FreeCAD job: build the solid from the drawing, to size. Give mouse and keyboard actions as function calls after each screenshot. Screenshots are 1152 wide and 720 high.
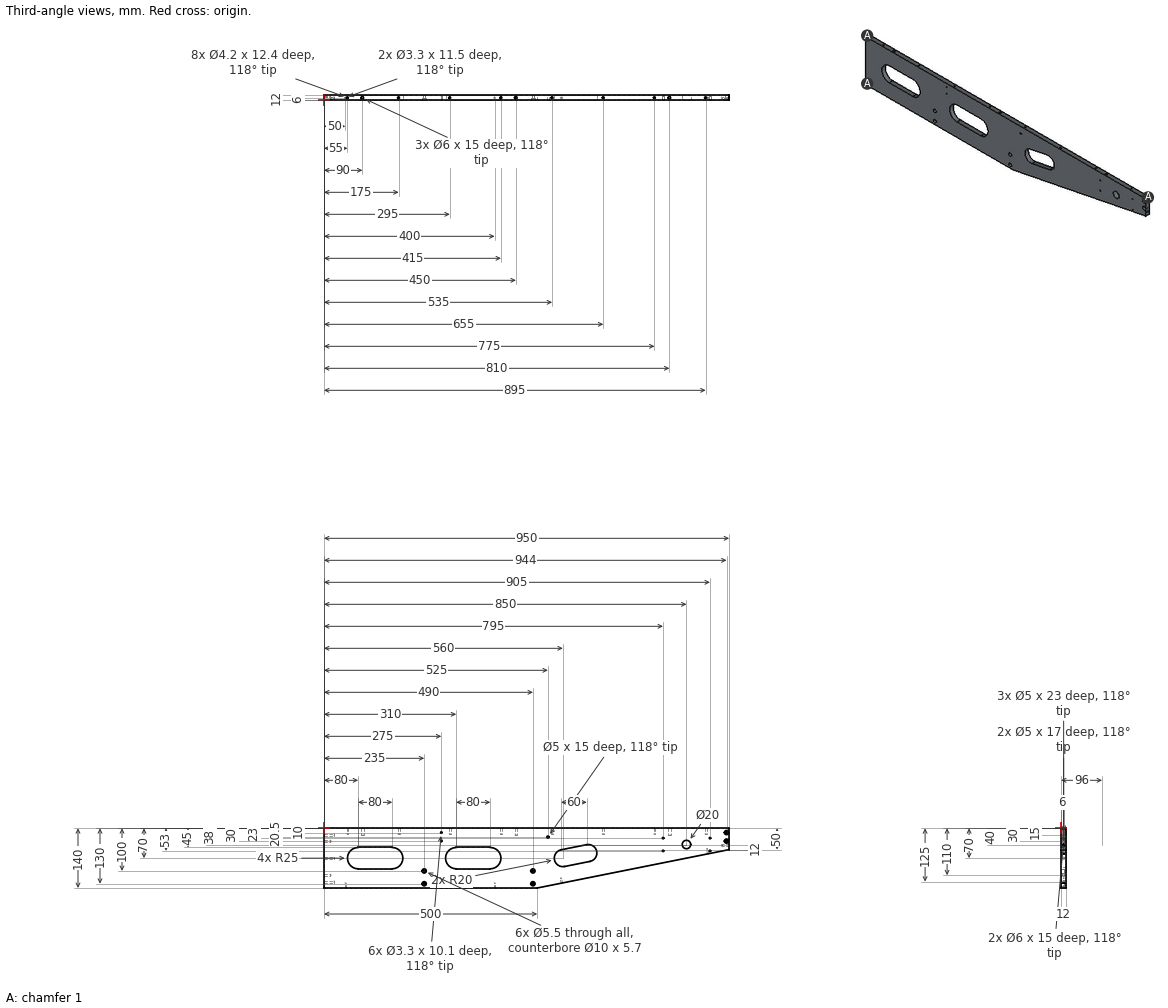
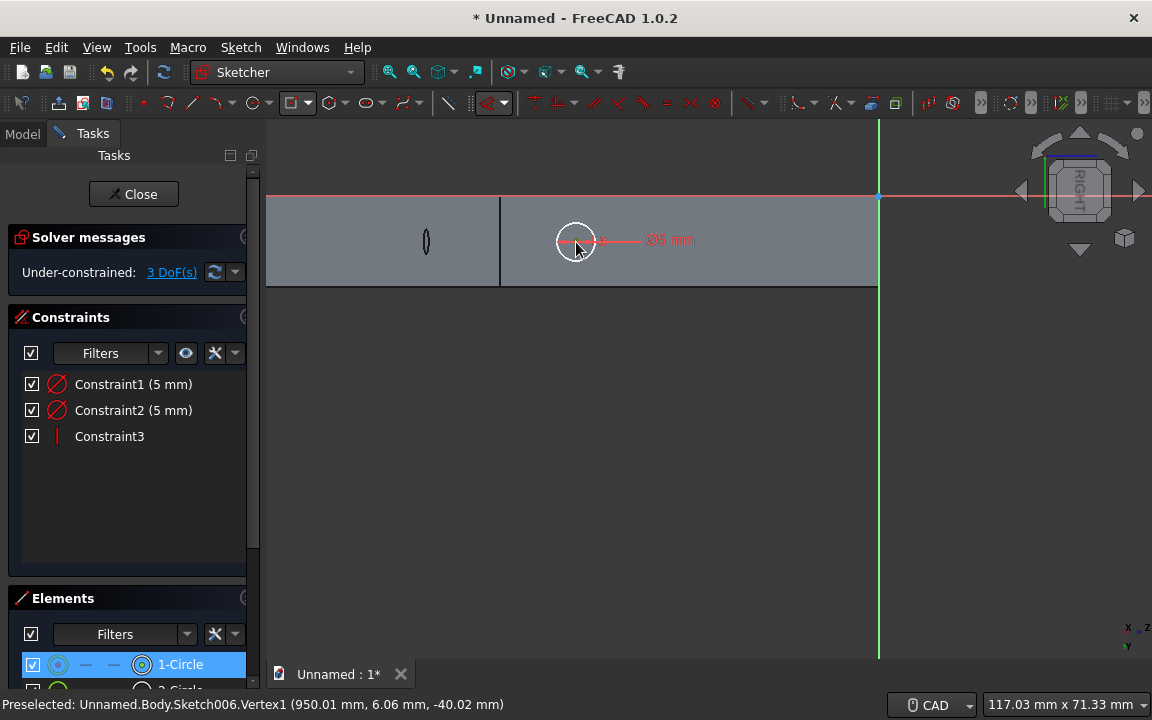
key(i)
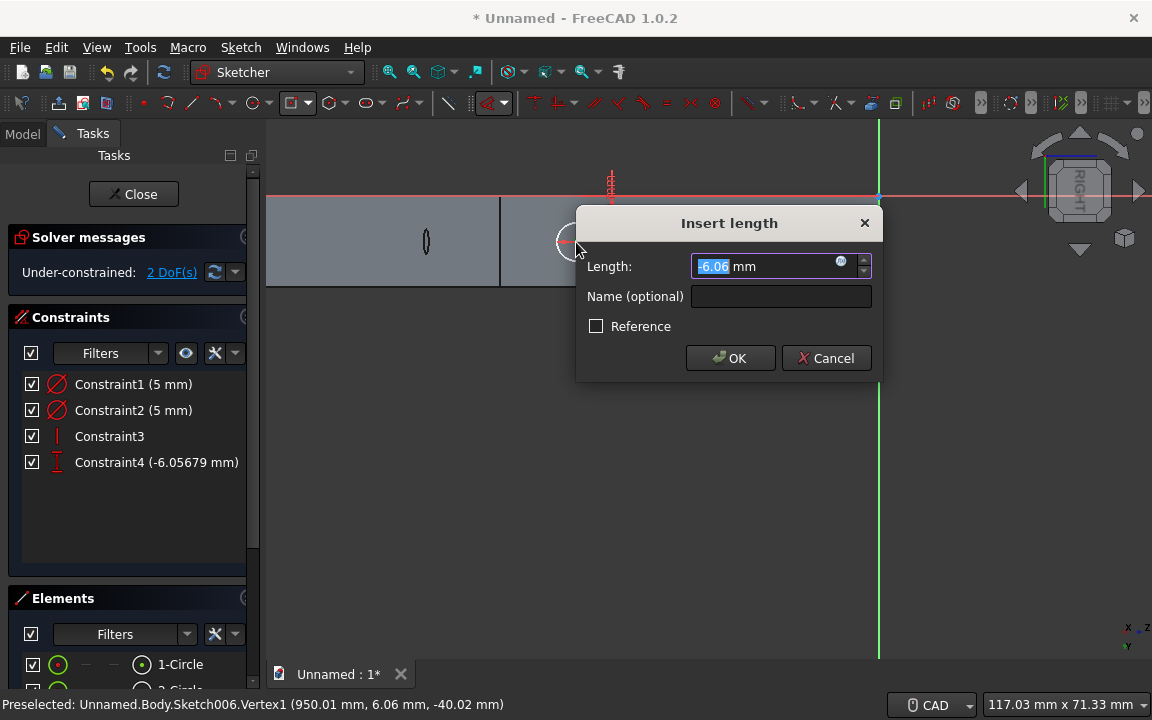
text(-6)
key(Return)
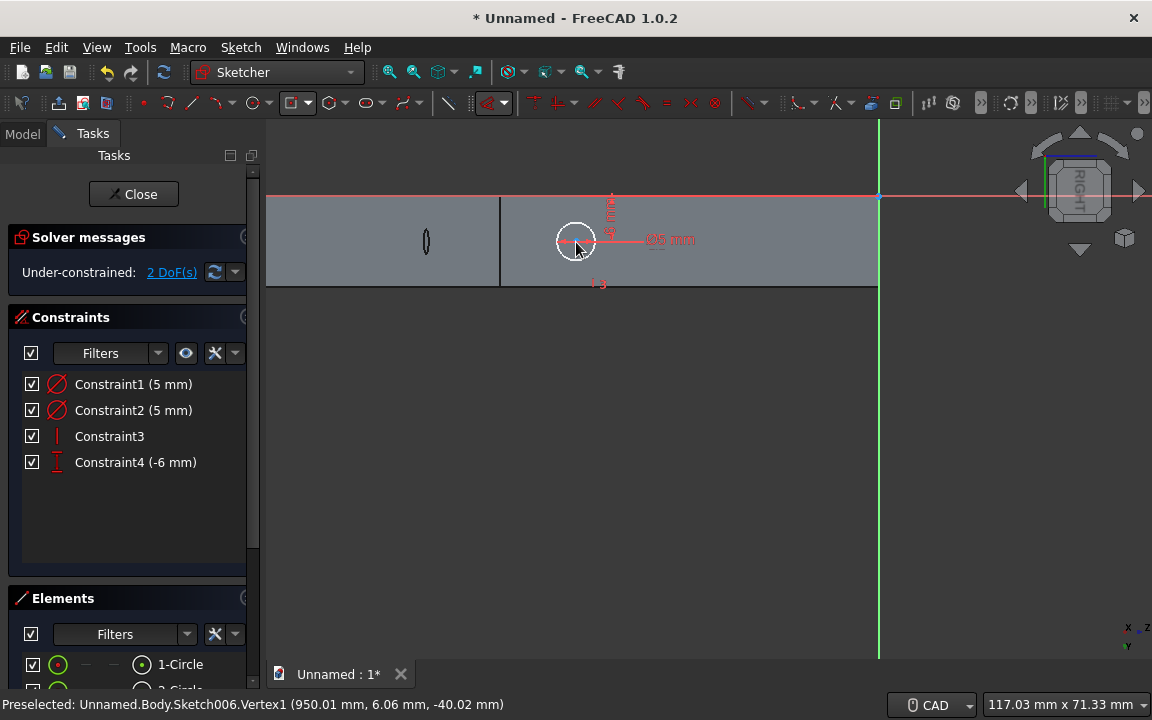
click(576, 242)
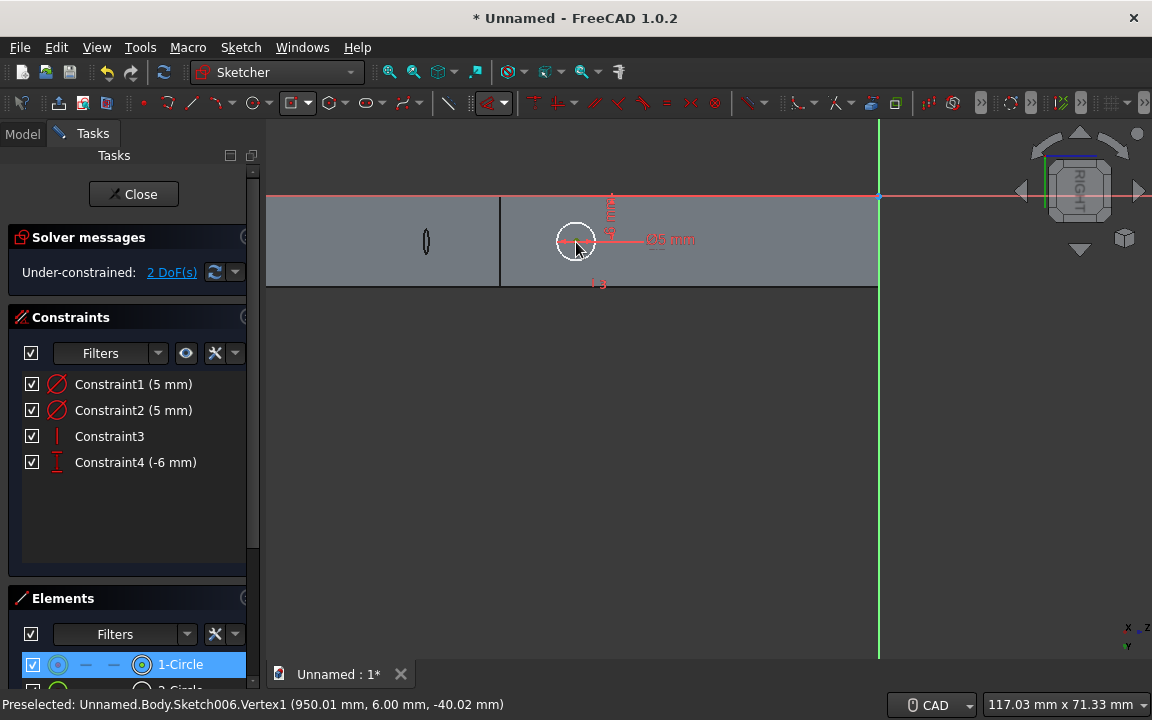
click(506, 104)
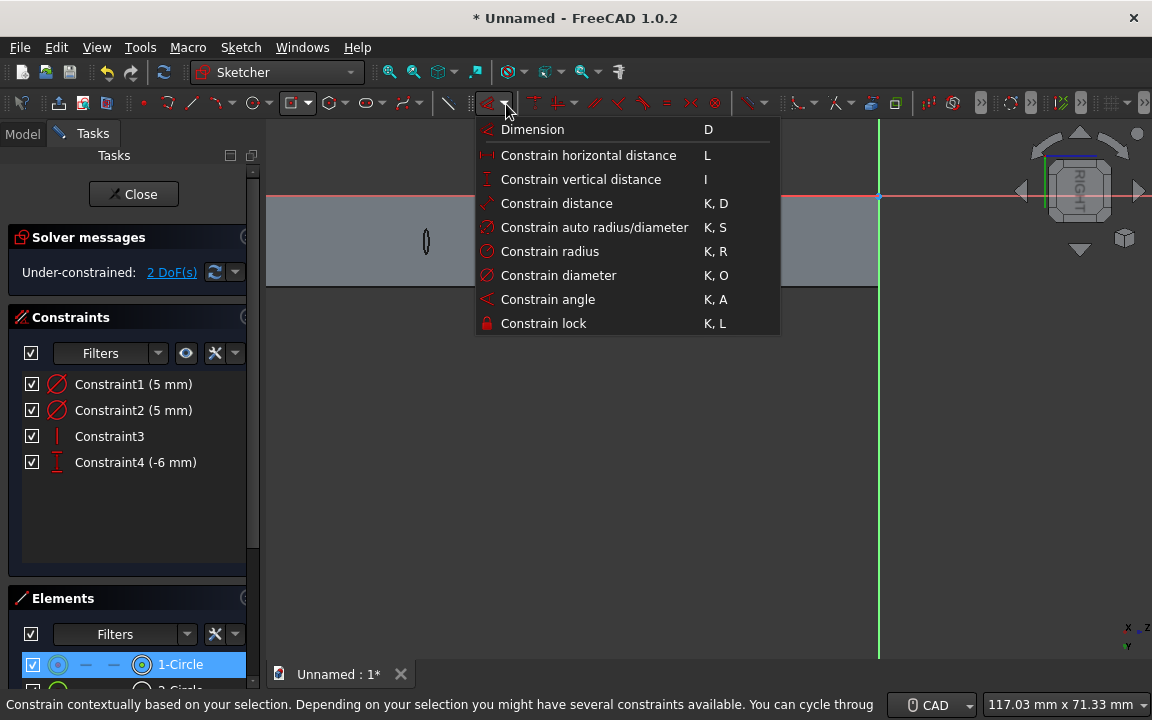
click(628, 155)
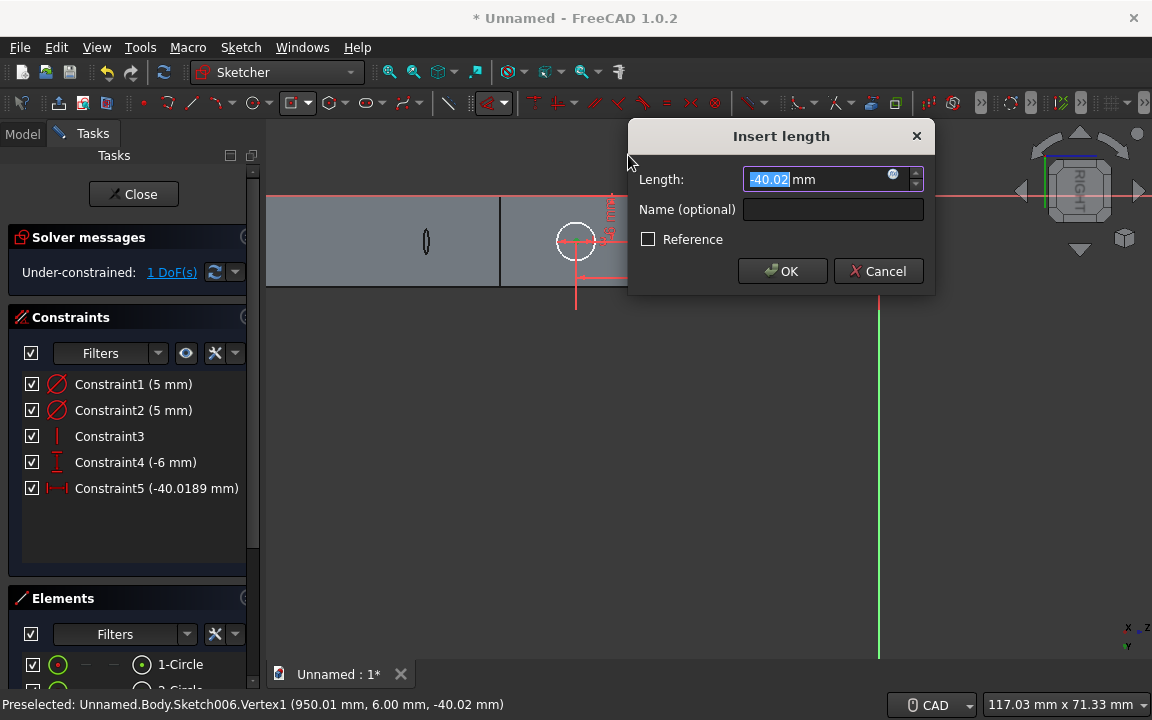
text(-40)
key(Return)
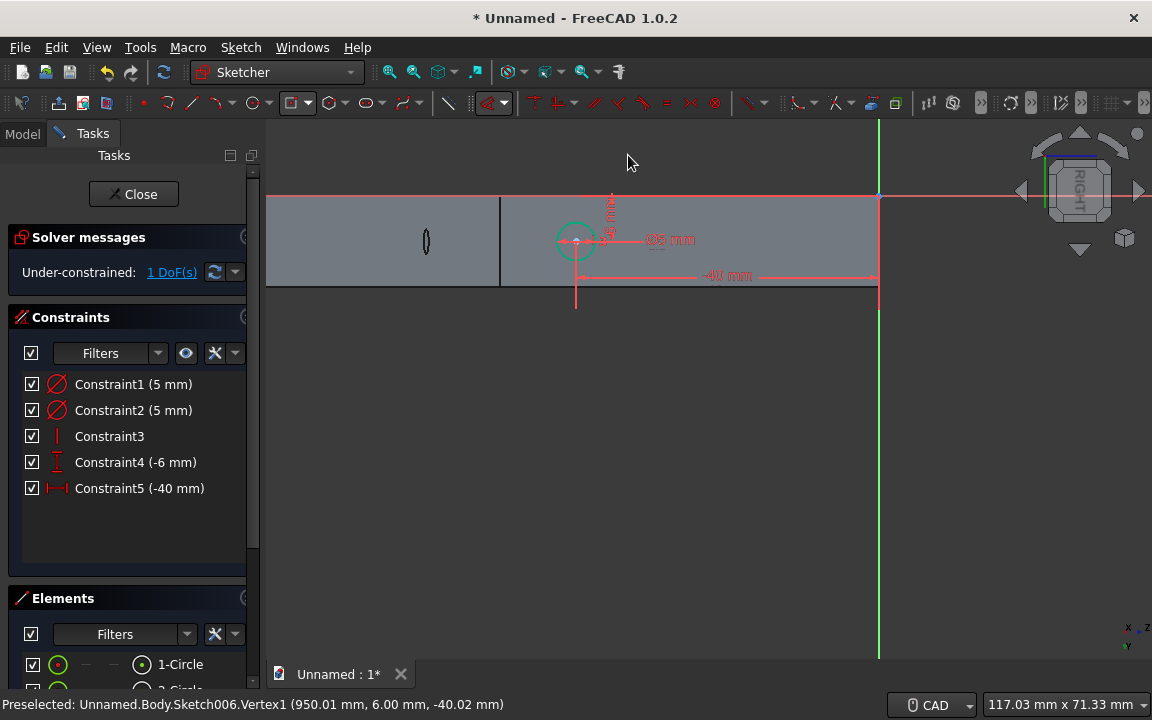
scroll(577, 242, down, 4)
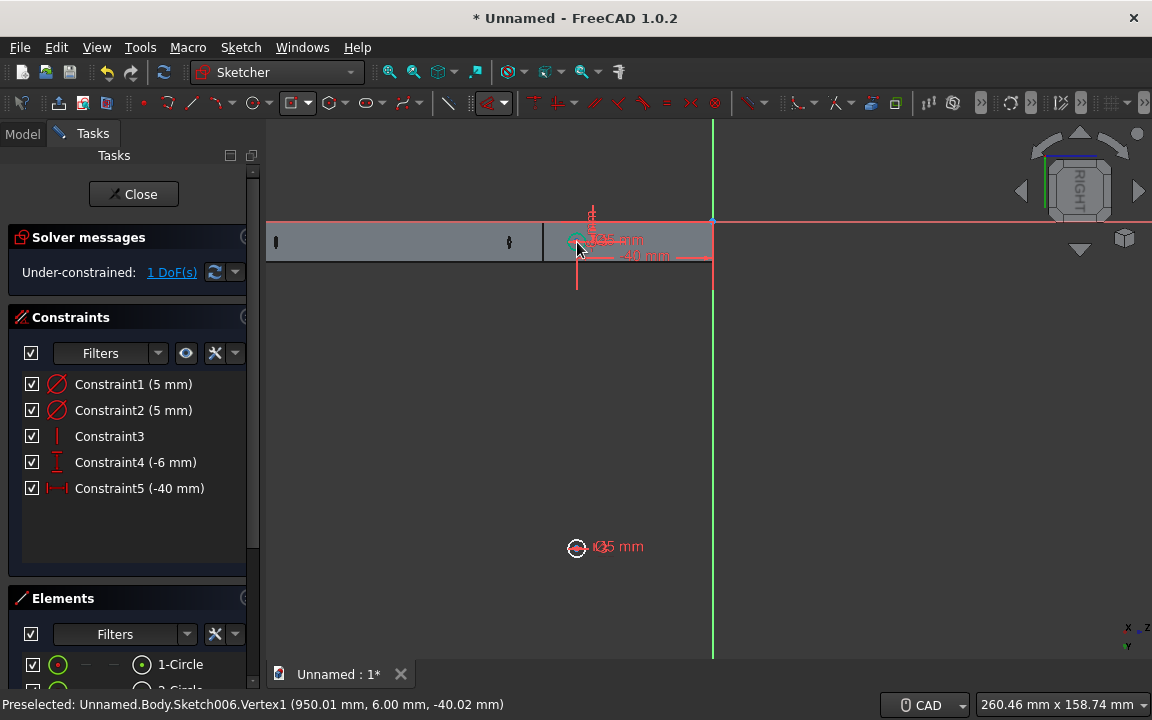
click(577, 549)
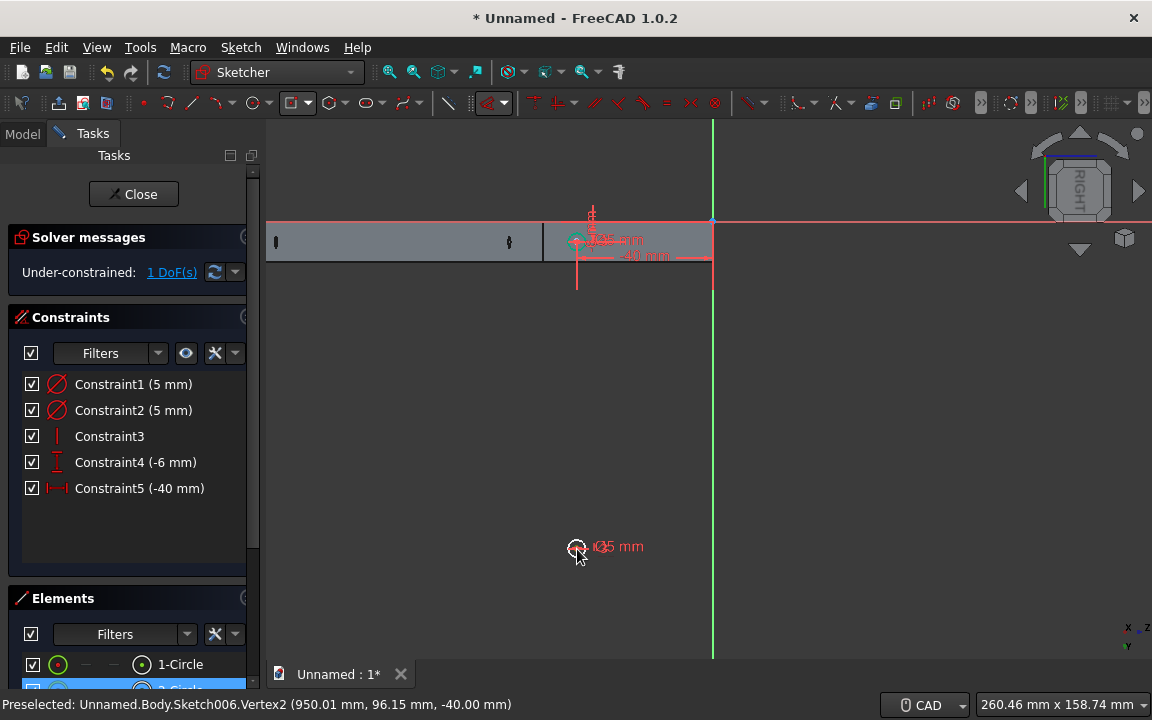
key(i)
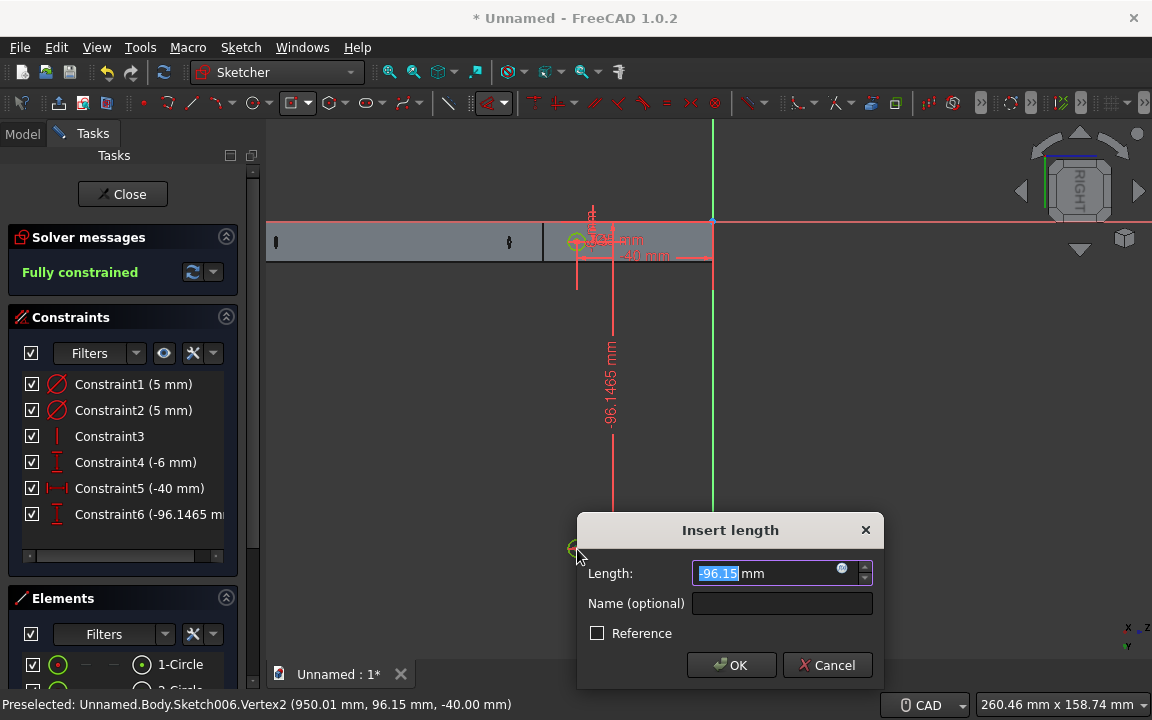
text(-96)
key(Return)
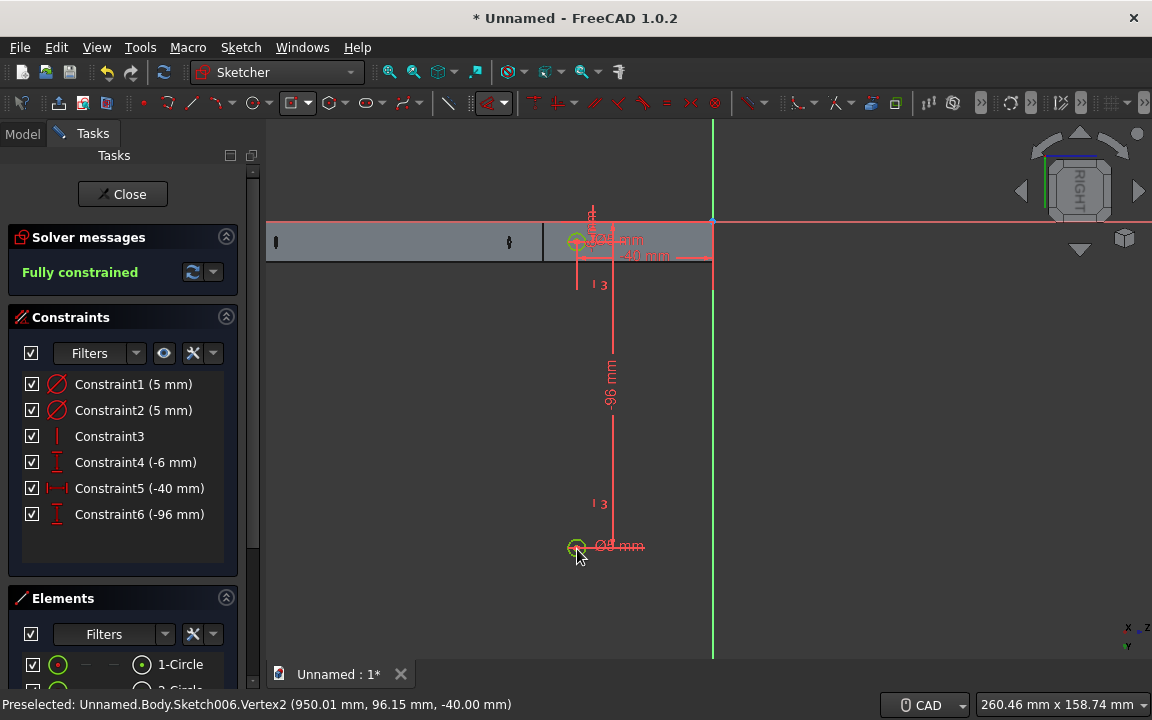
click(123, 194)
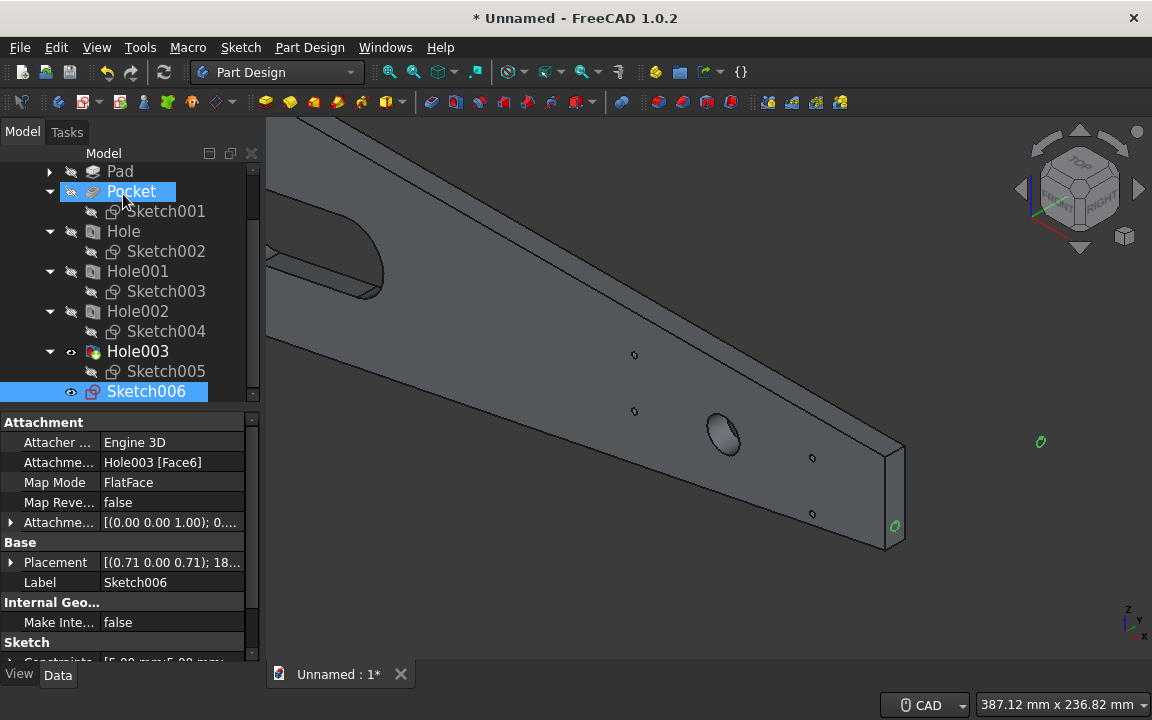
click(456, 102)